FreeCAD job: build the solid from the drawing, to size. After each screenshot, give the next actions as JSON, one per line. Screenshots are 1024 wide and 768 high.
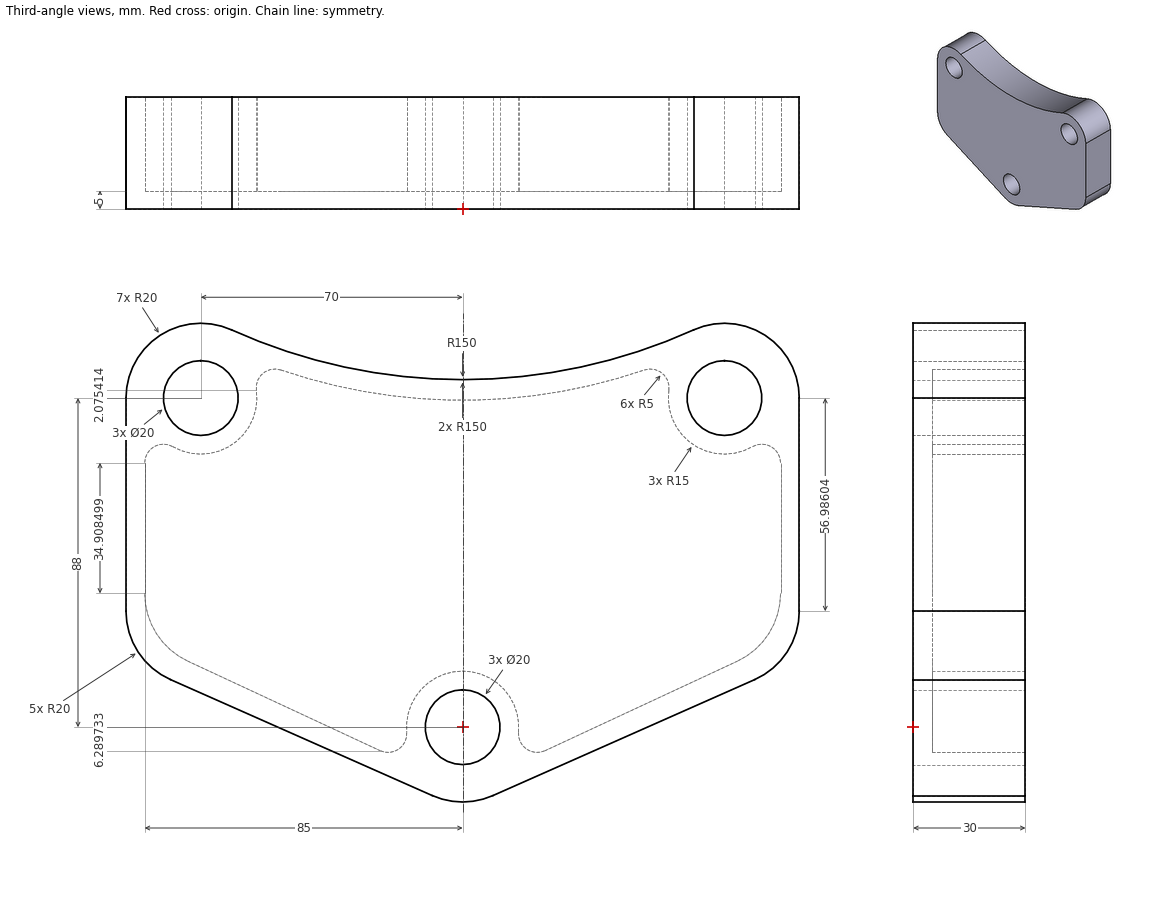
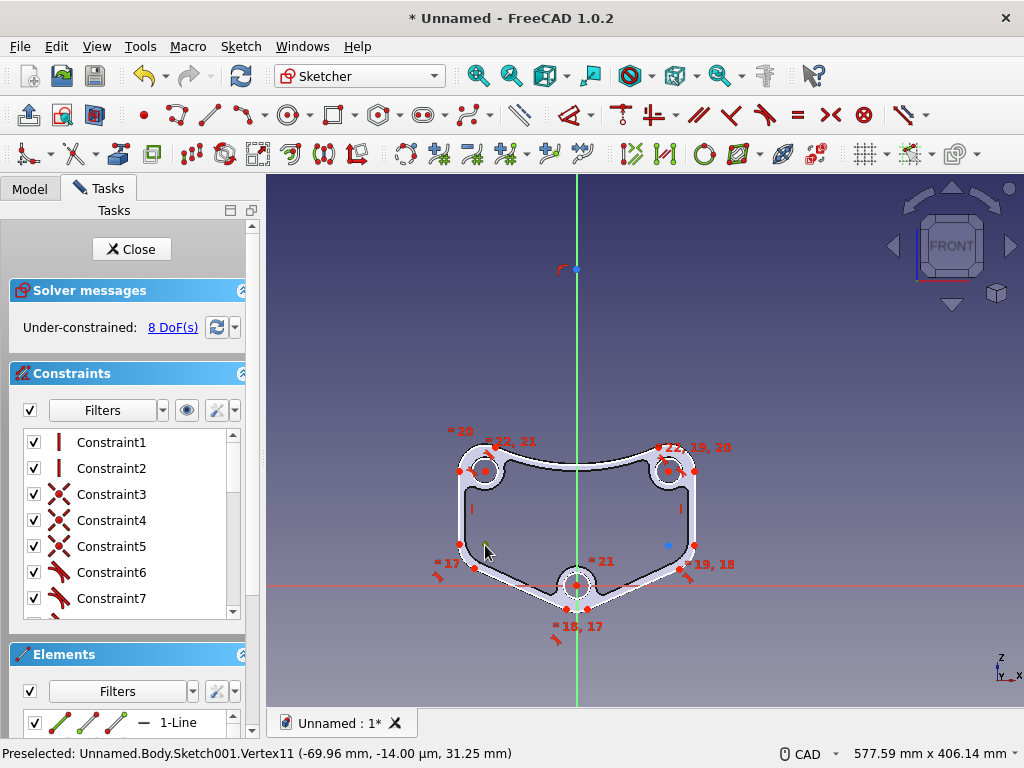
{"action": "left_click", "coordinate": [669, 546]}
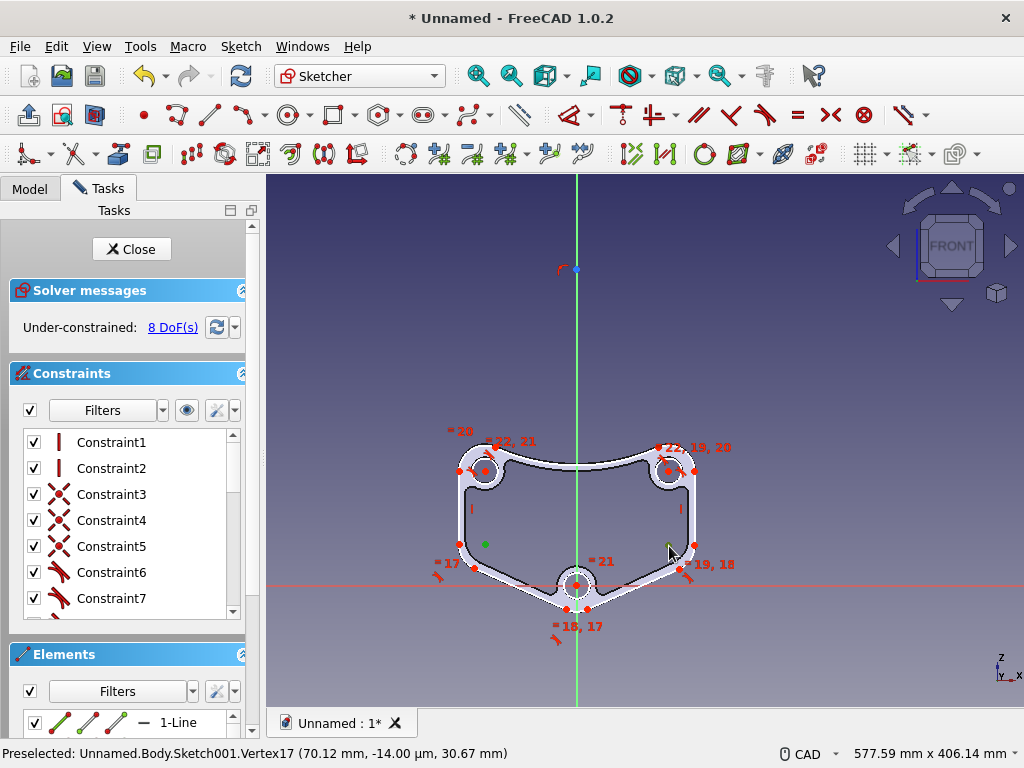
{"action": "left_click", "coordinate": [577, 543]}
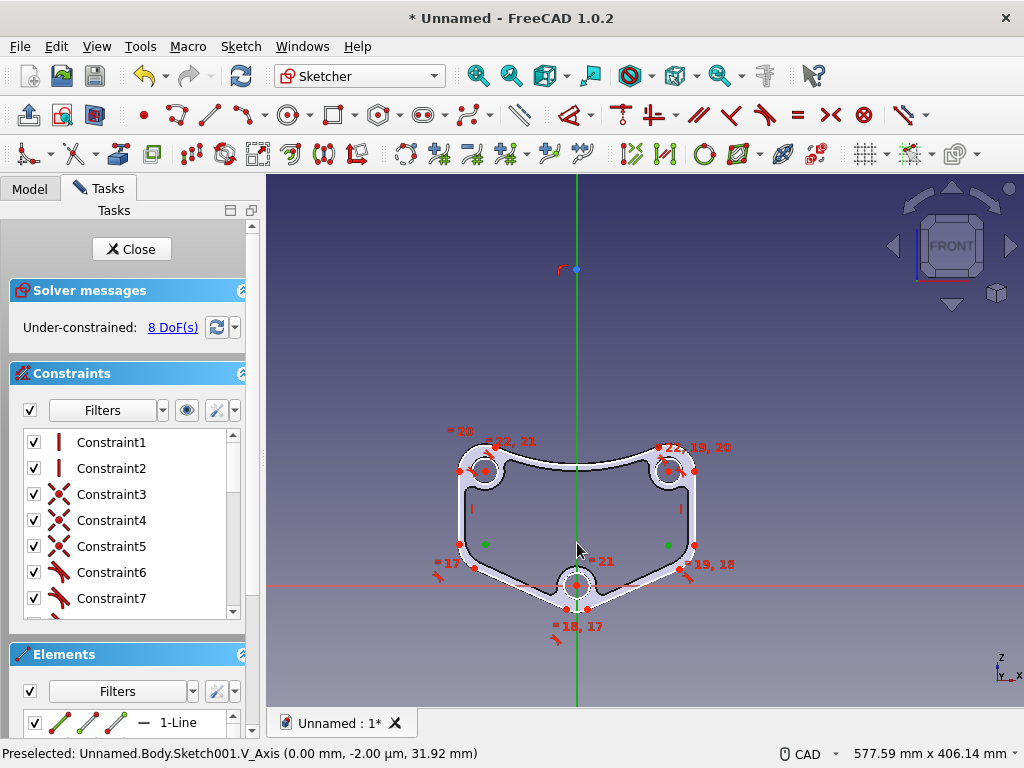
{"action": "left_click", "coordinate": [831, 116]}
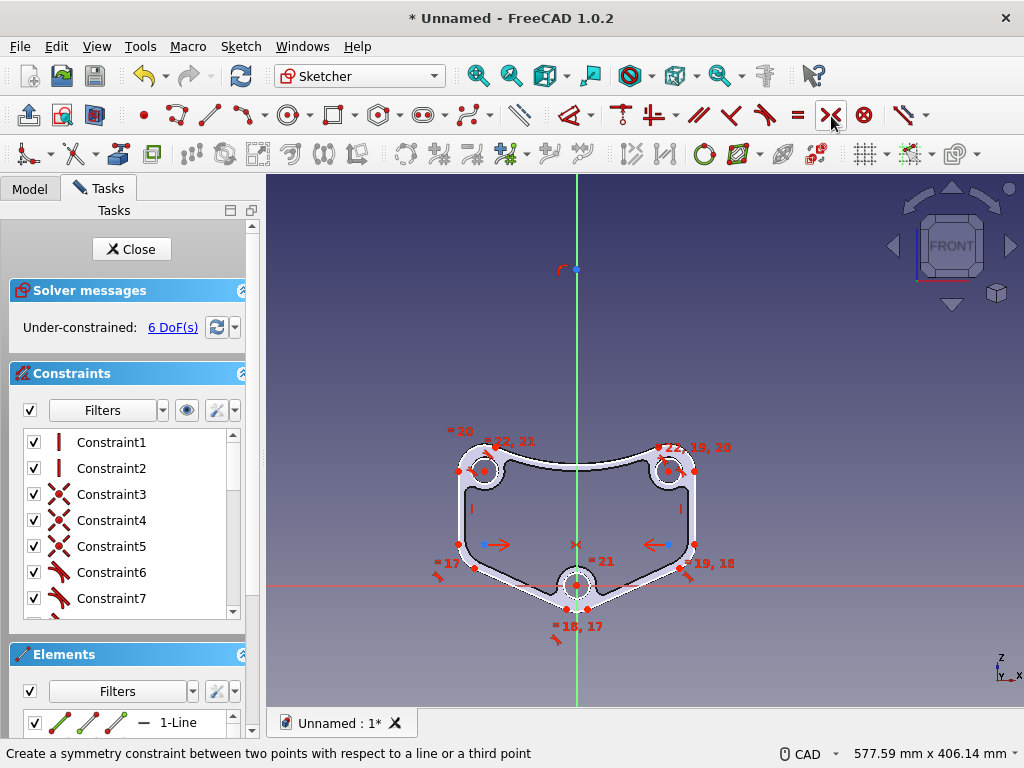
{"action": "key", "text": "d"}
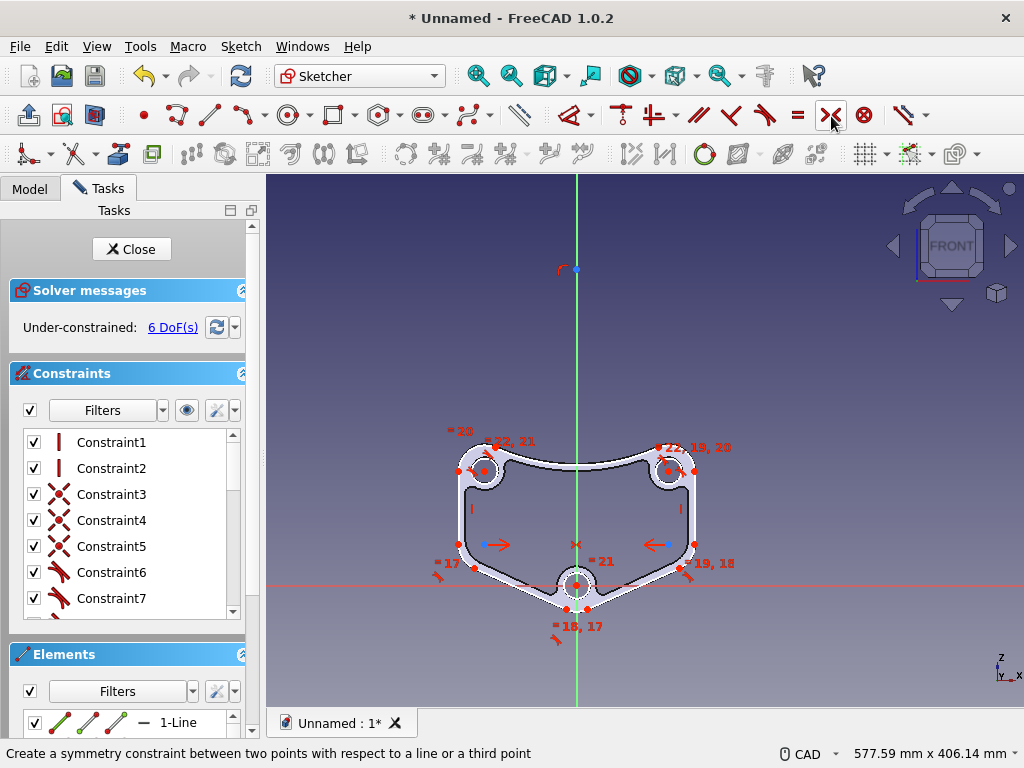
{"action": "scroll", "coordinate": [463, 559], "scroll_direction": "up", "scroll_amount": 3}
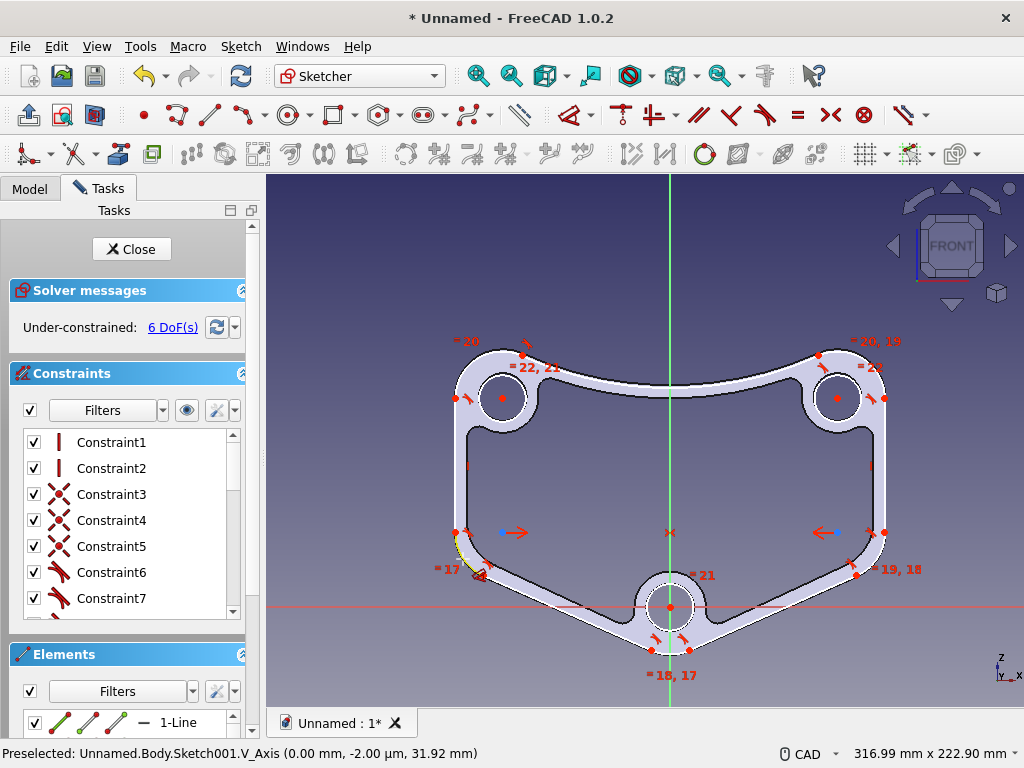
{"action": "left_click", "coordinate": [463, 558]}
{"action": "left_click", "coordinate": [436, 575]}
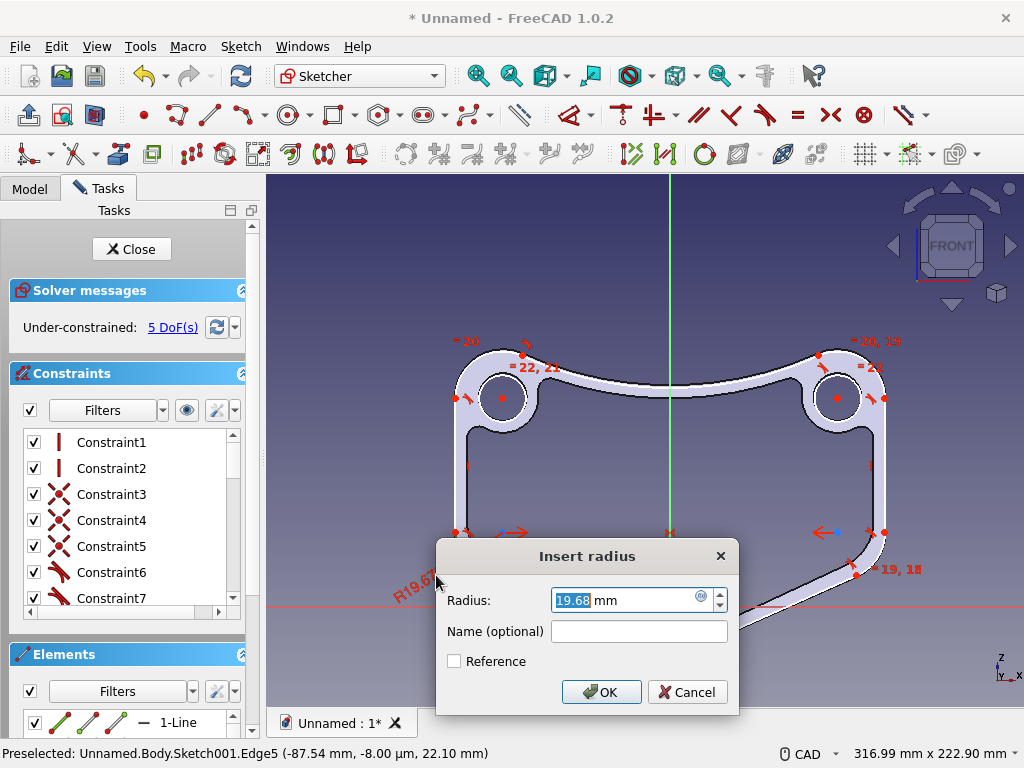
{"action": "type", "text": "20"}
{"action": "key", "text": "Return"}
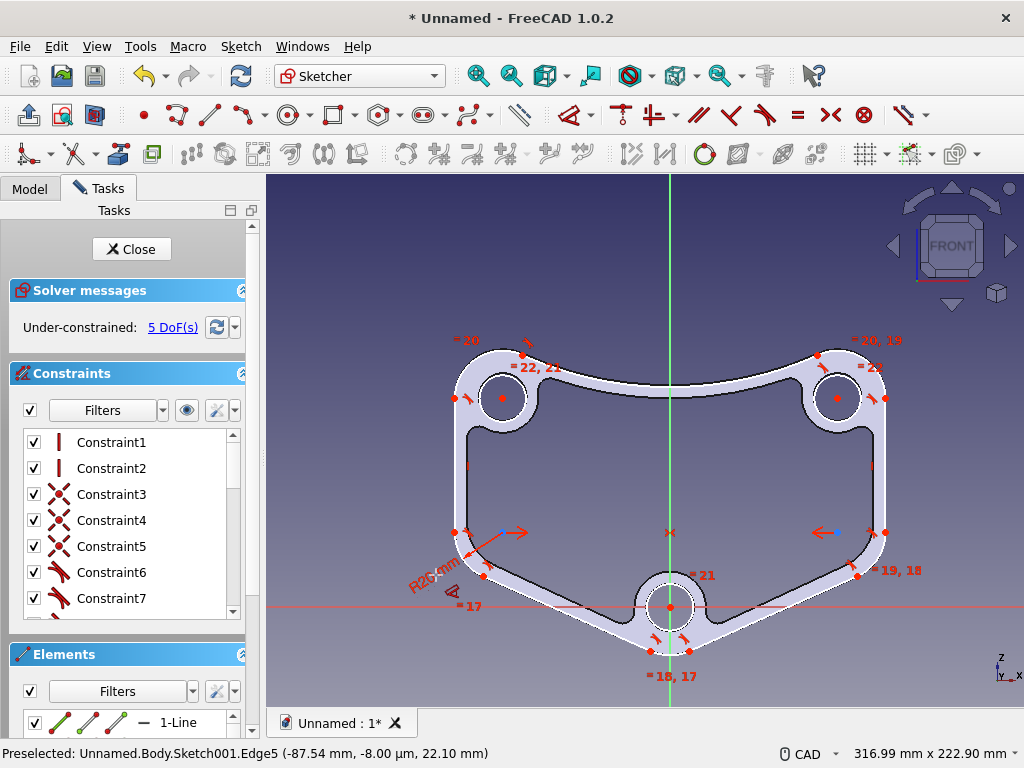
{"action": "left_click", "coordinate": [610, 382]}
{"action": "left_click", "coordinate": [605, 414]}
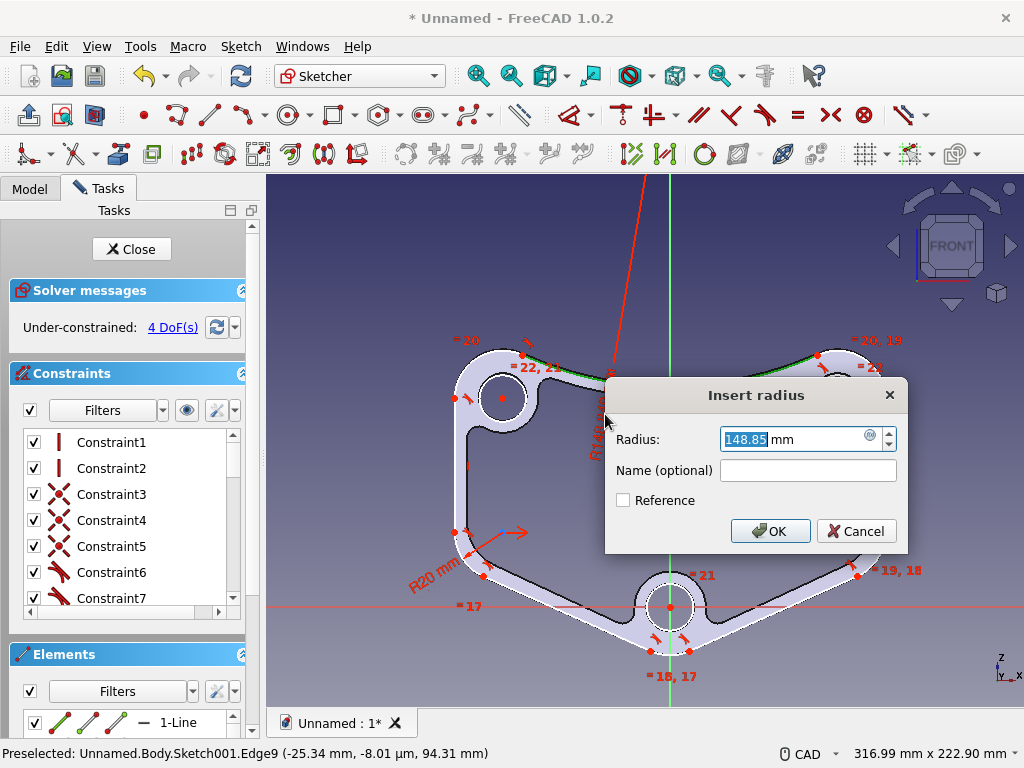
{"action": "type", "text": "150"}
{"action": "key", "text": "Return"}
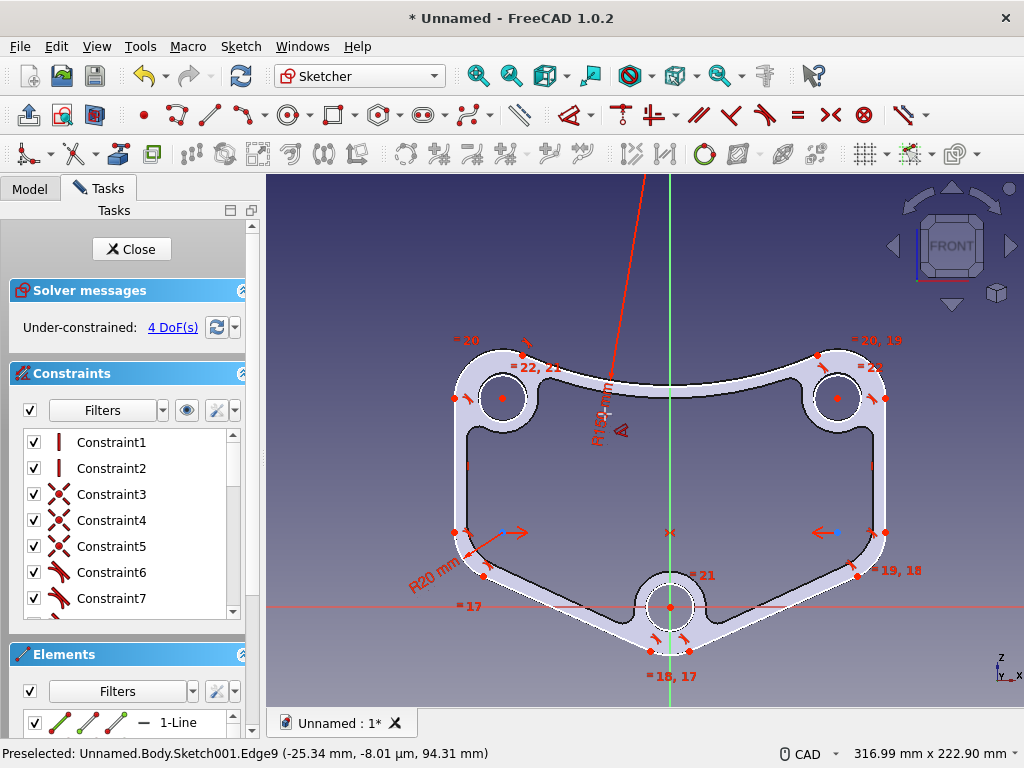
{"action": "left_click", "coordinate": [687, 591]}
{"action": "left_click", "coordinate": [710, 569]}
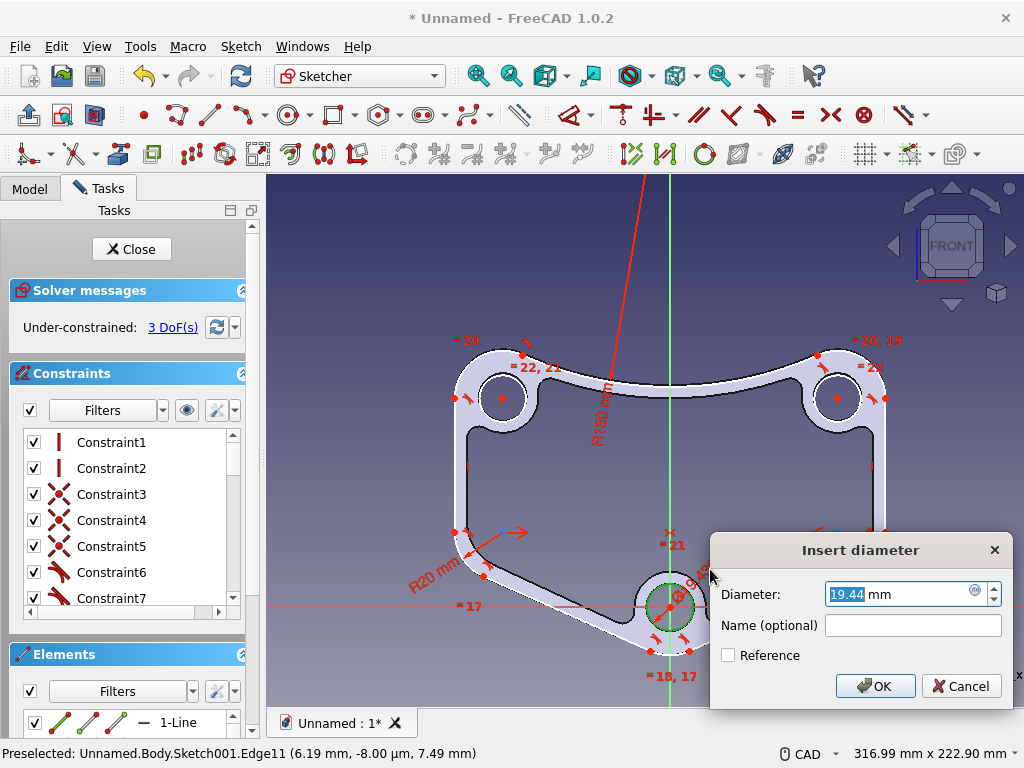
{"action": "type", "text": "20"}
{"action": "key", "text": "Return"}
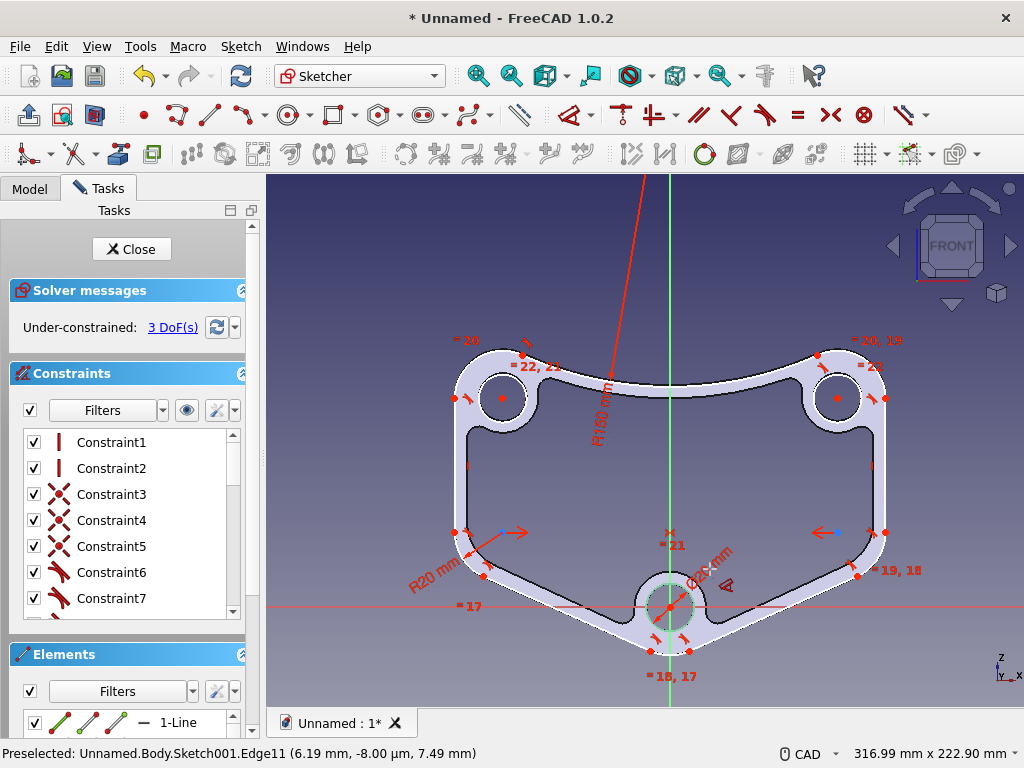
{"action": "left_click", "coordinate": [503, 399]}
{"action": "left_click", "coordinate": [625, 365]}